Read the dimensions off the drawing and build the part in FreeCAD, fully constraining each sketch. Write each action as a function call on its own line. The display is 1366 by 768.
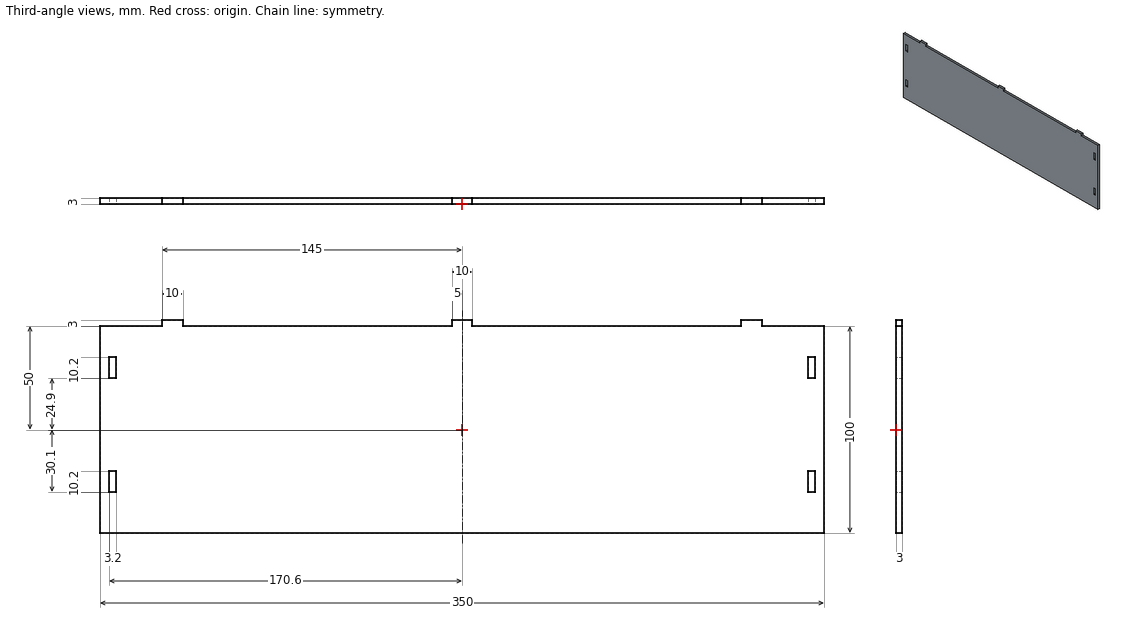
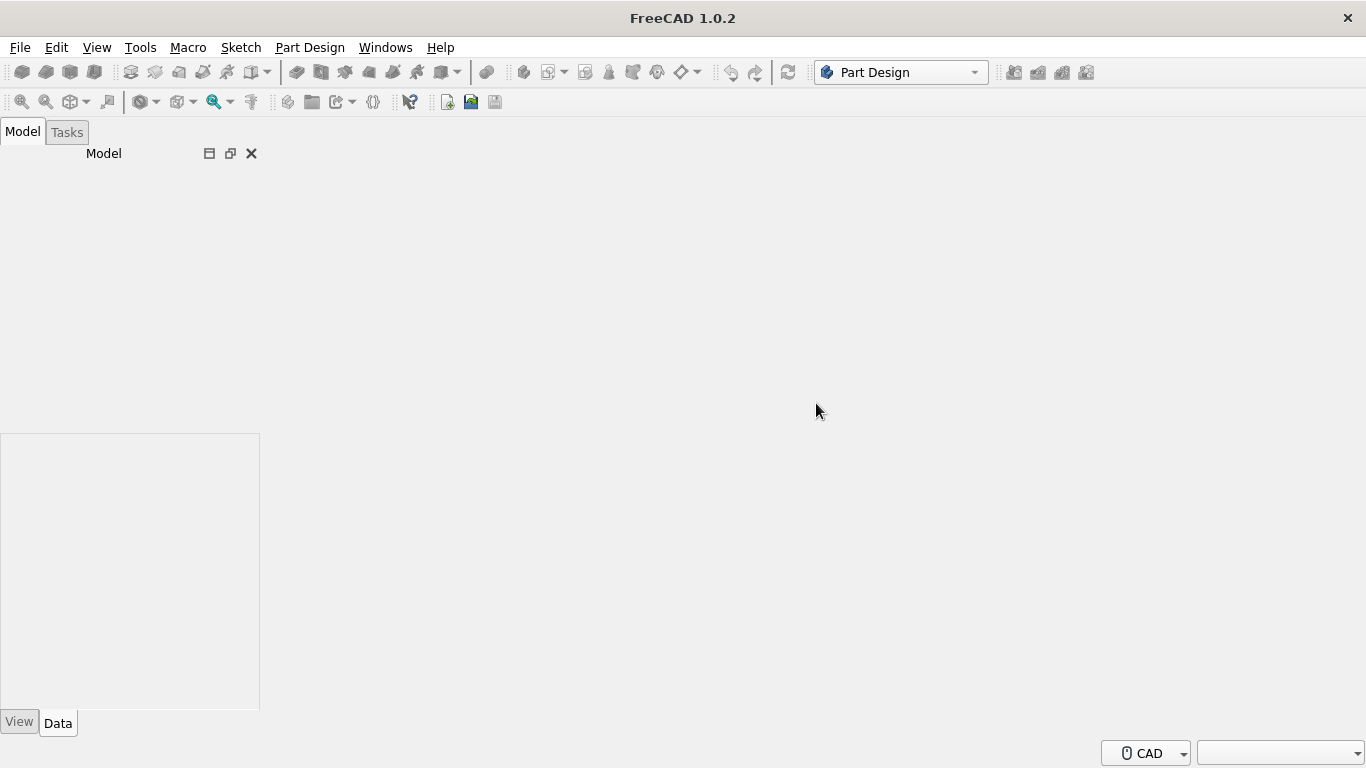
key(ctrl+n)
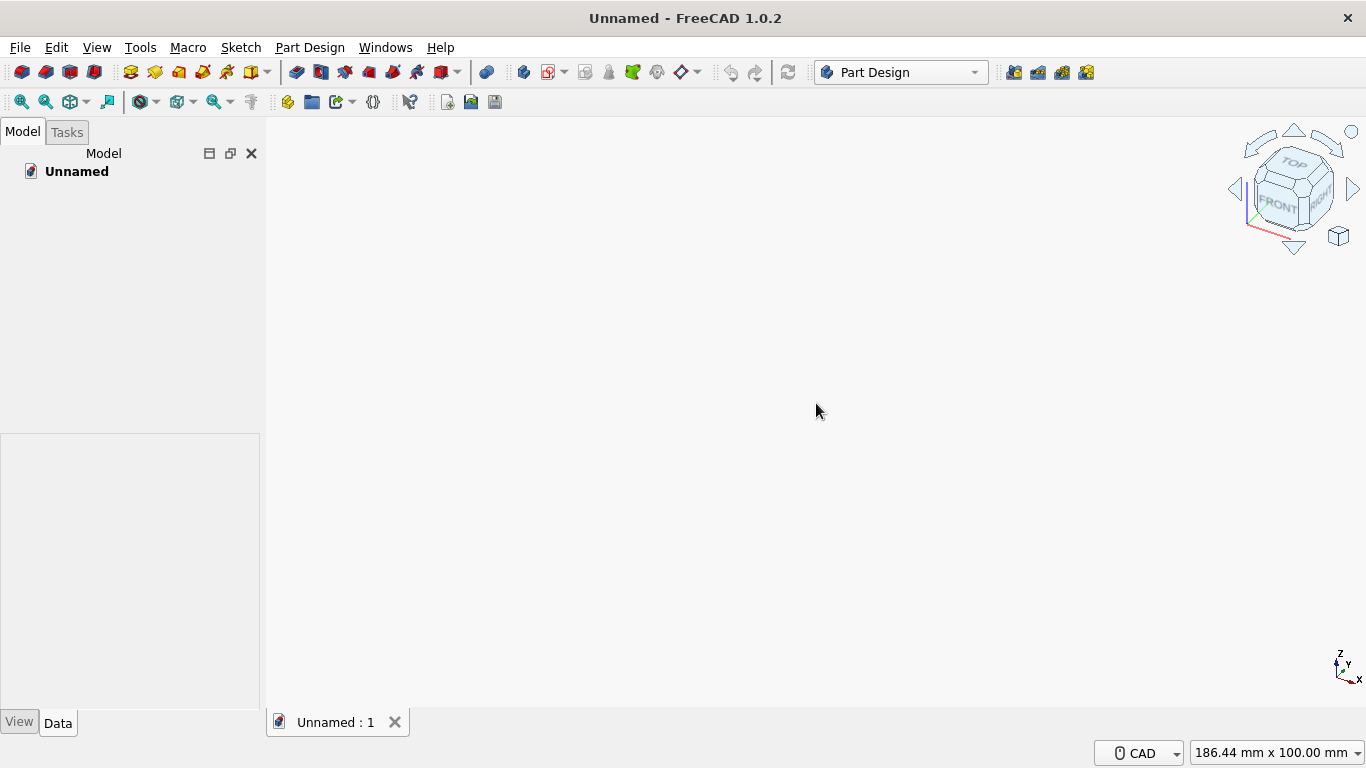
click(548, 72)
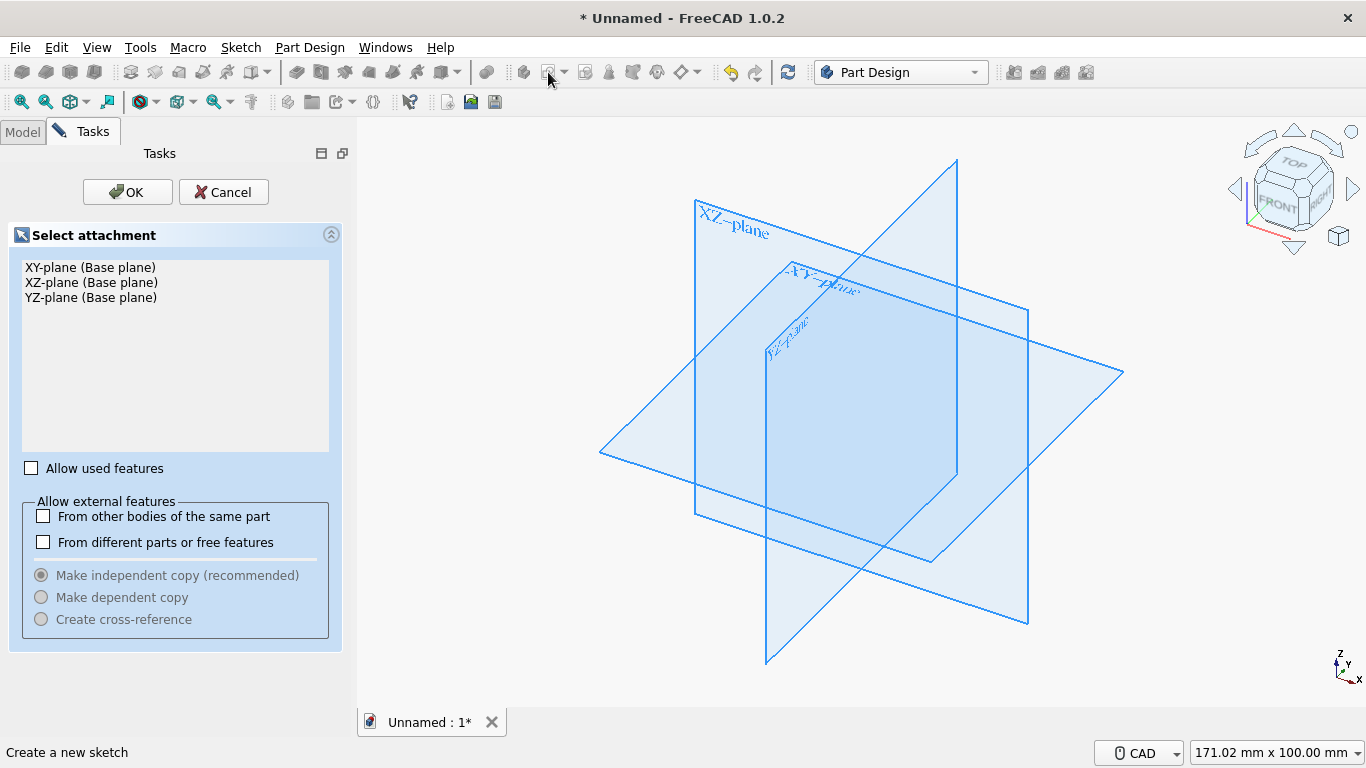
click(82, 282)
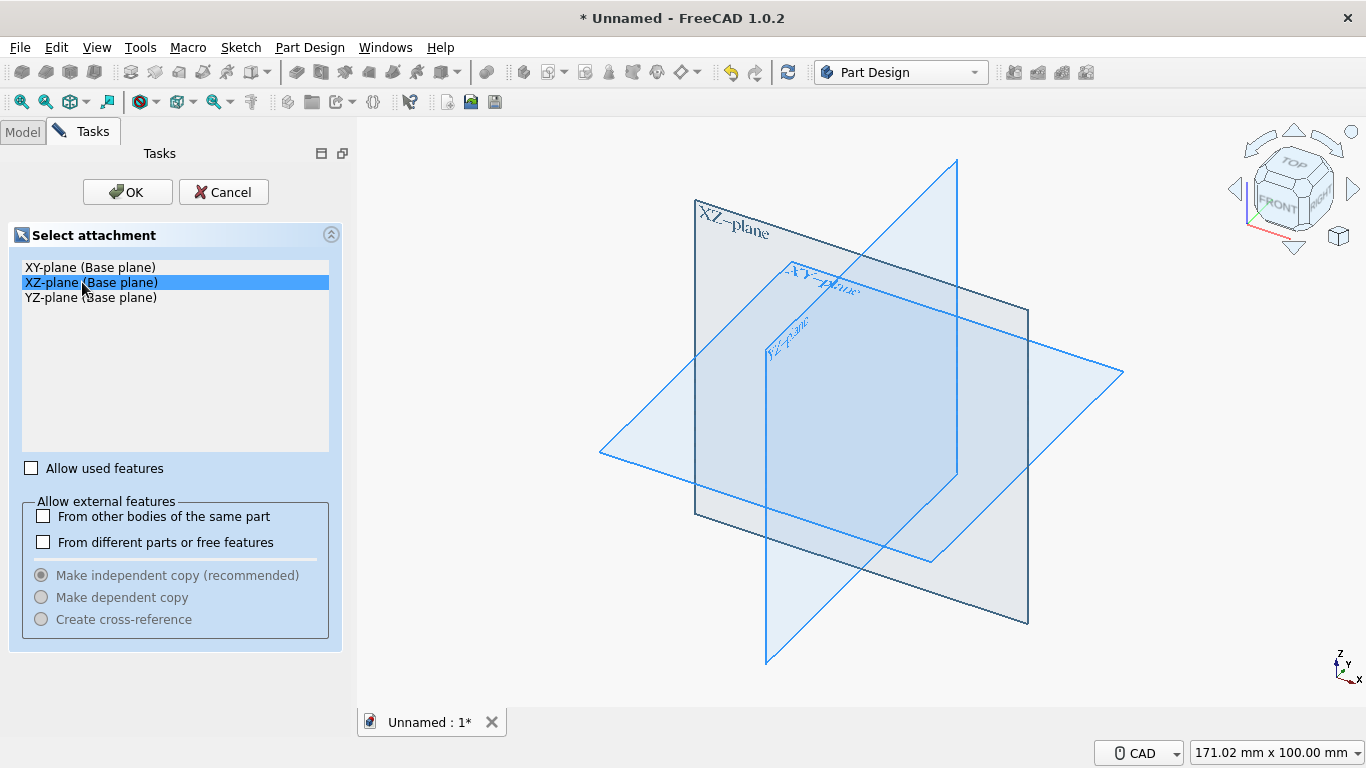
click(128, 192)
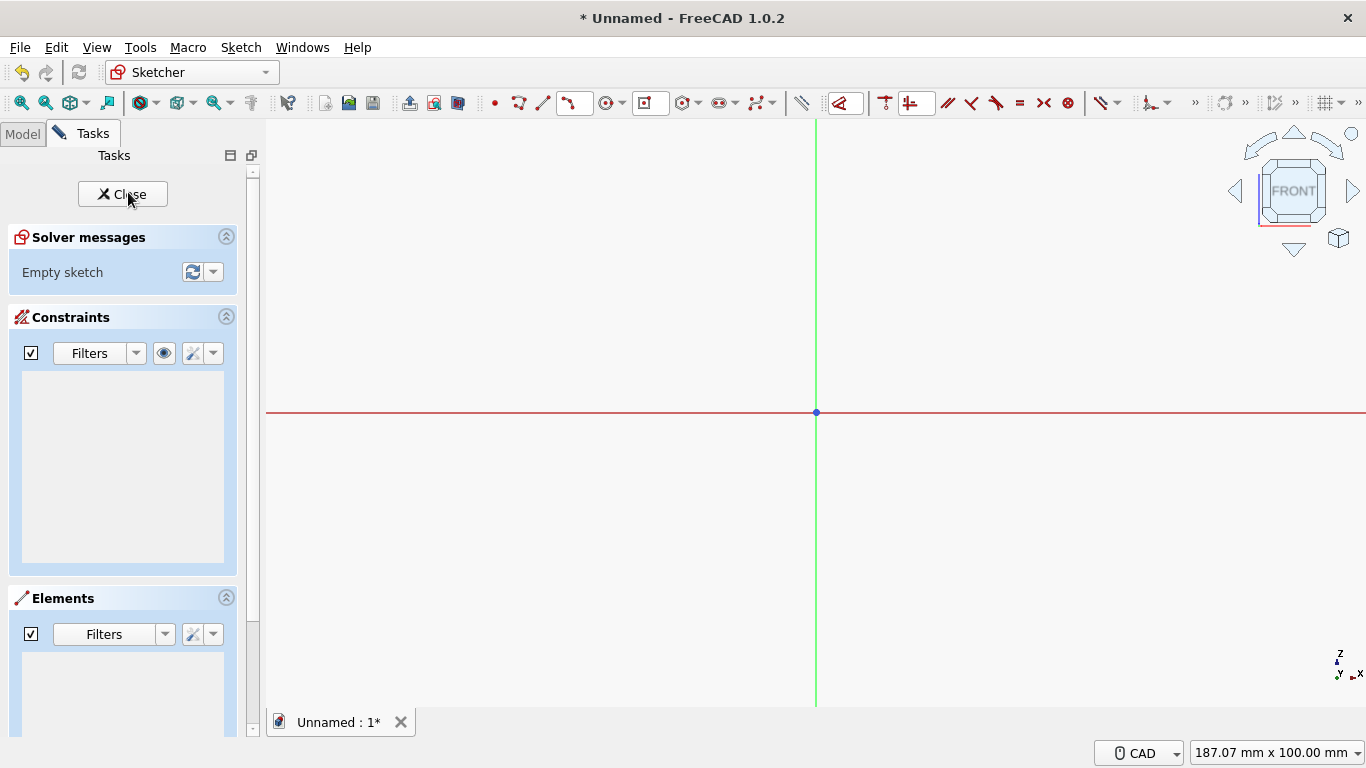
scroll(718, 413, down, 6)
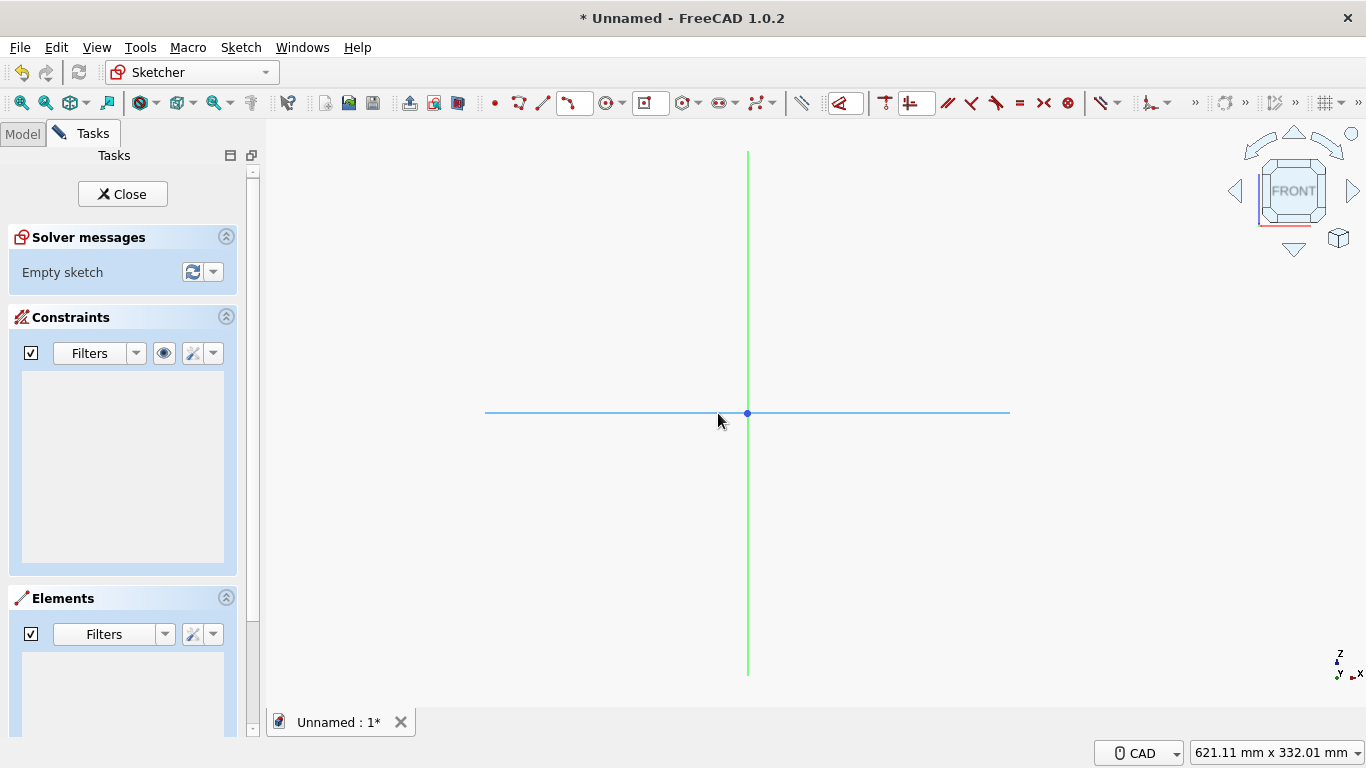
key(g)
key(v)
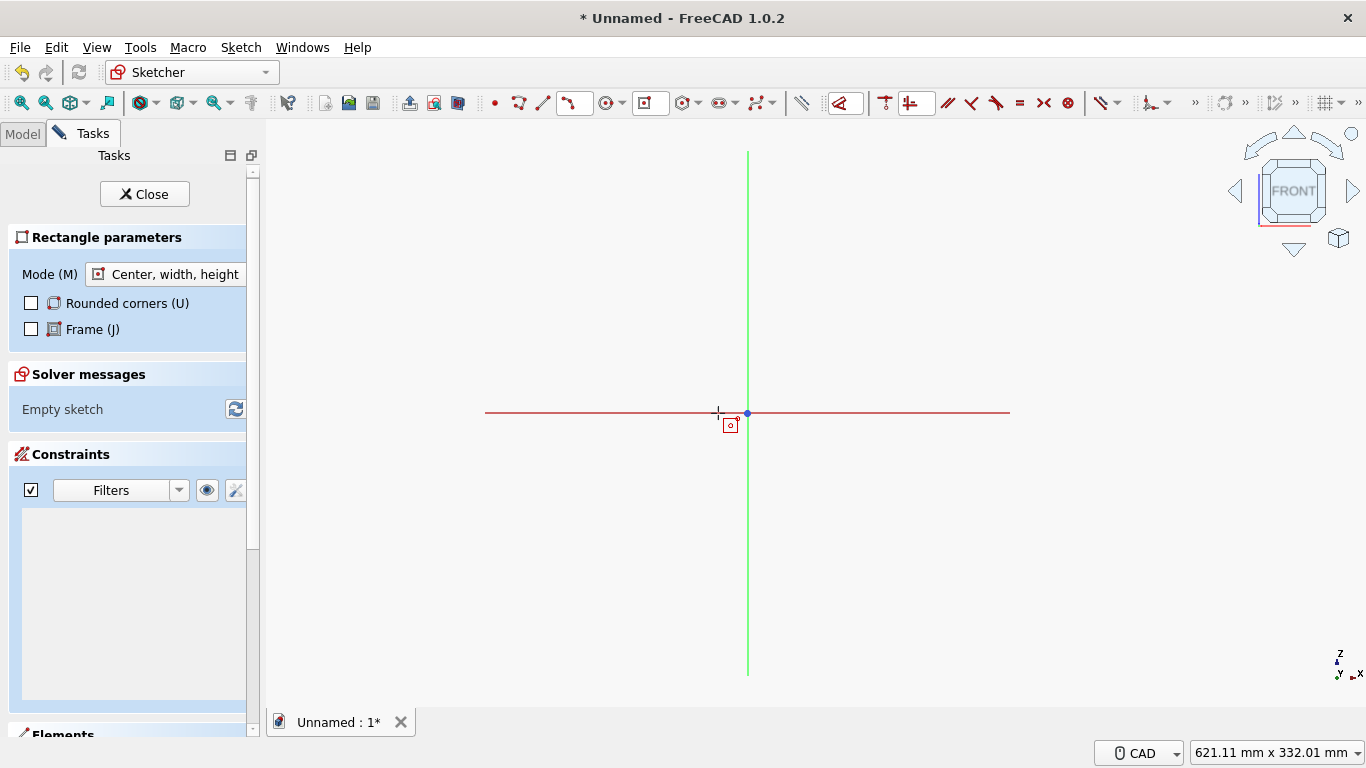
click(748, 413)
click(1058, 325)
key(Escape)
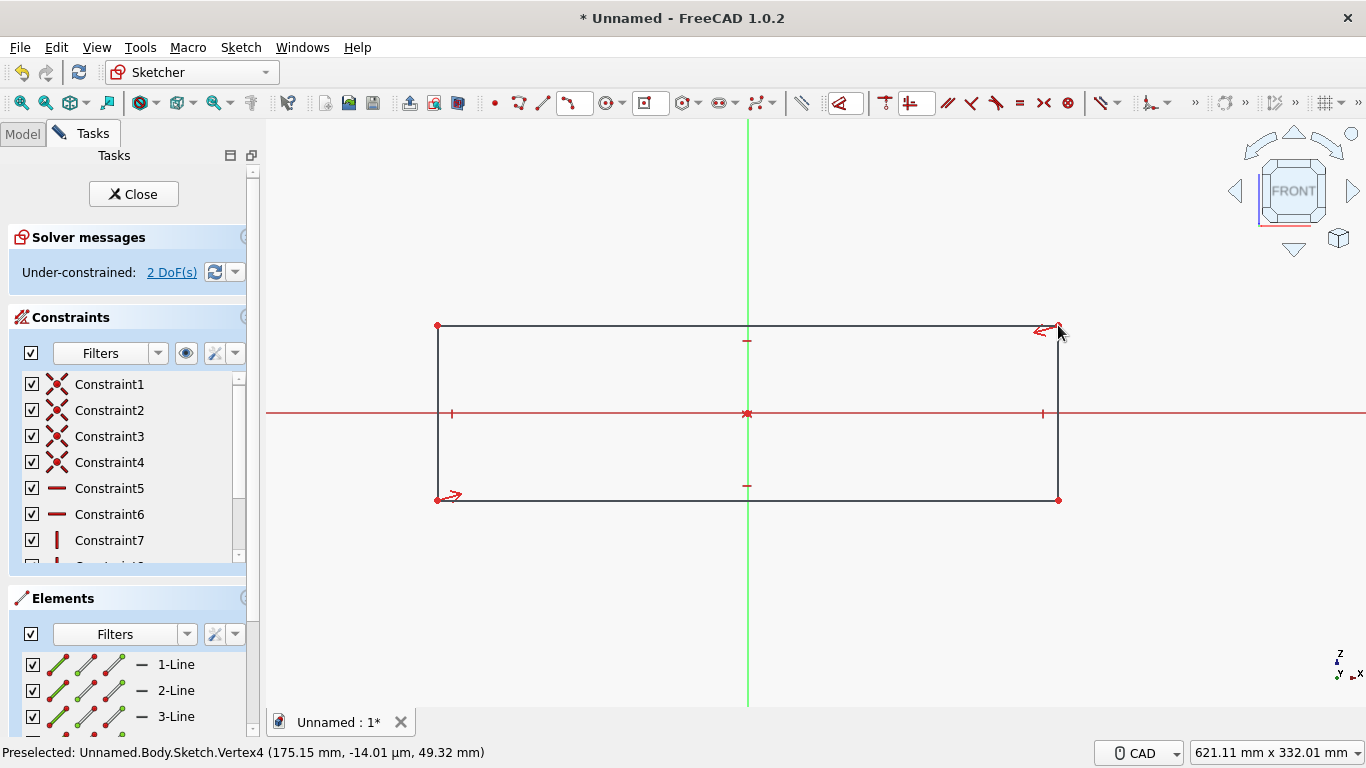
key(d)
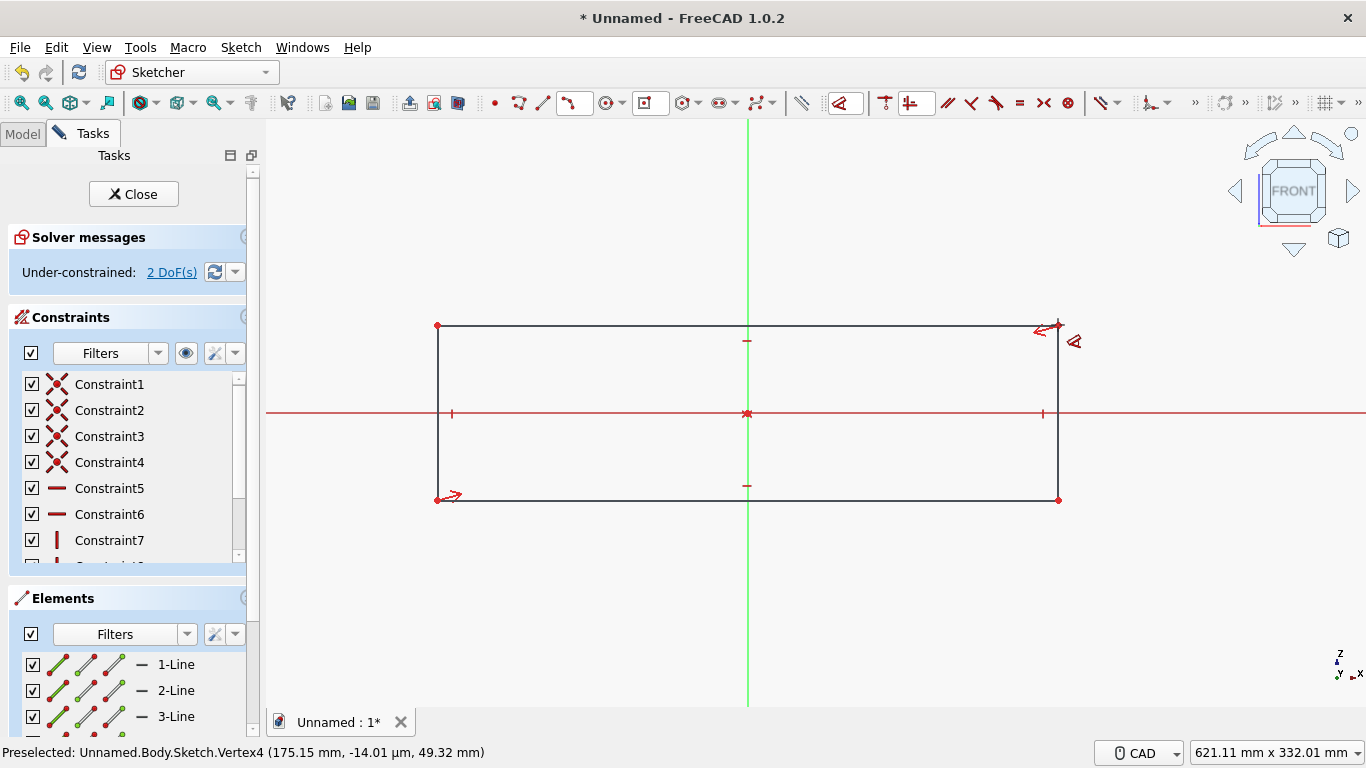
click(624, 501)
click(605, 535)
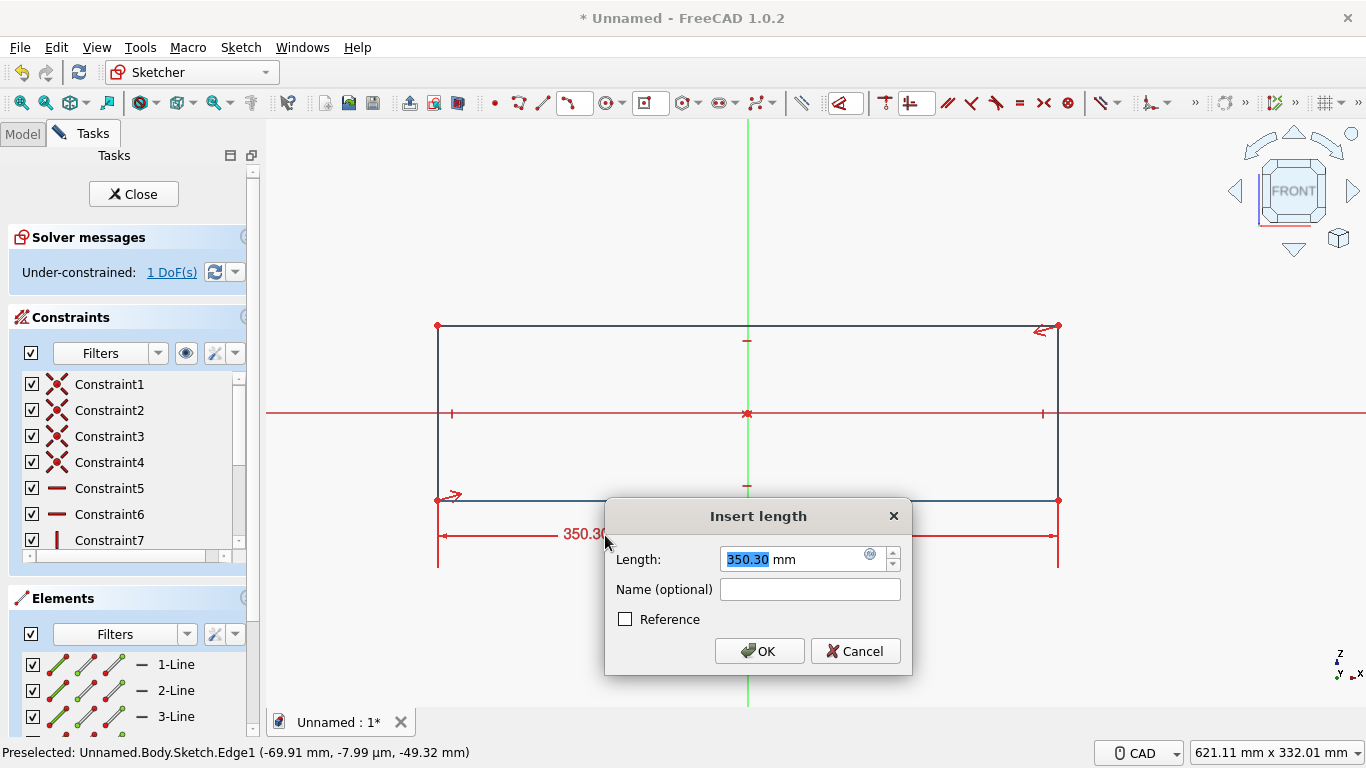
text(350)
key(Return)